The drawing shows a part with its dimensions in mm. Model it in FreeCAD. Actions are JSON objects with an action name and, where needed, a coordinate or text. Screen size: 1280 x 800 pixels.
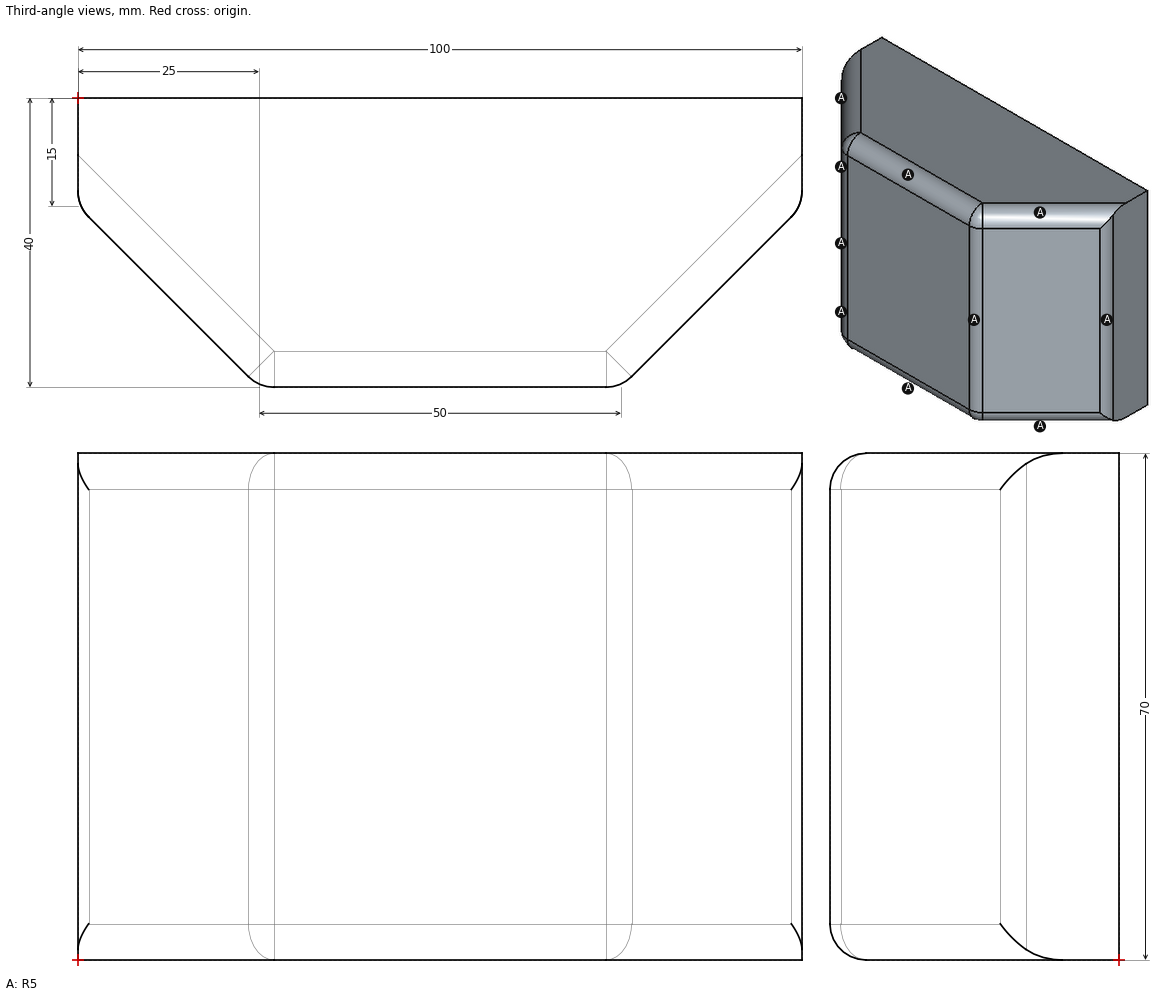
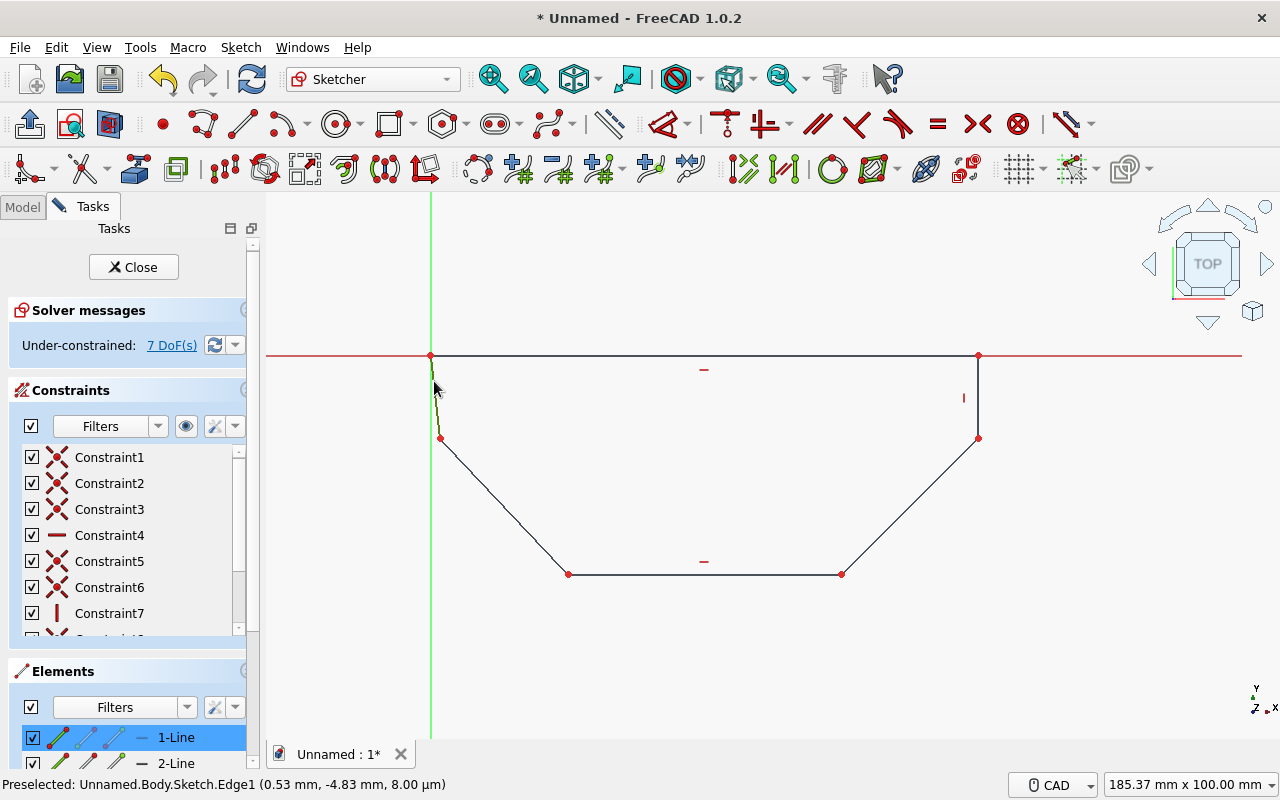
{"action": "left_click", "coordinate": [792, 124]}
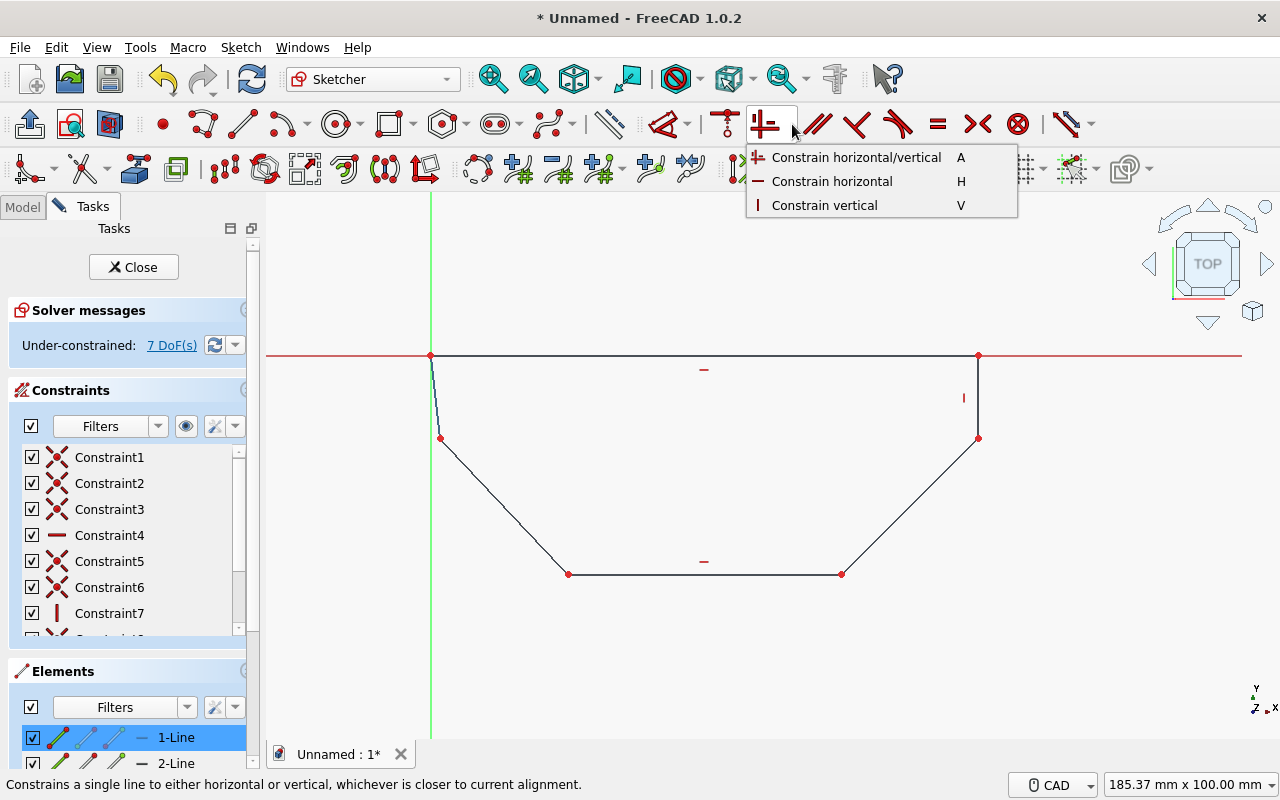
{"action": "left_click", "coordinate": [882, 205]}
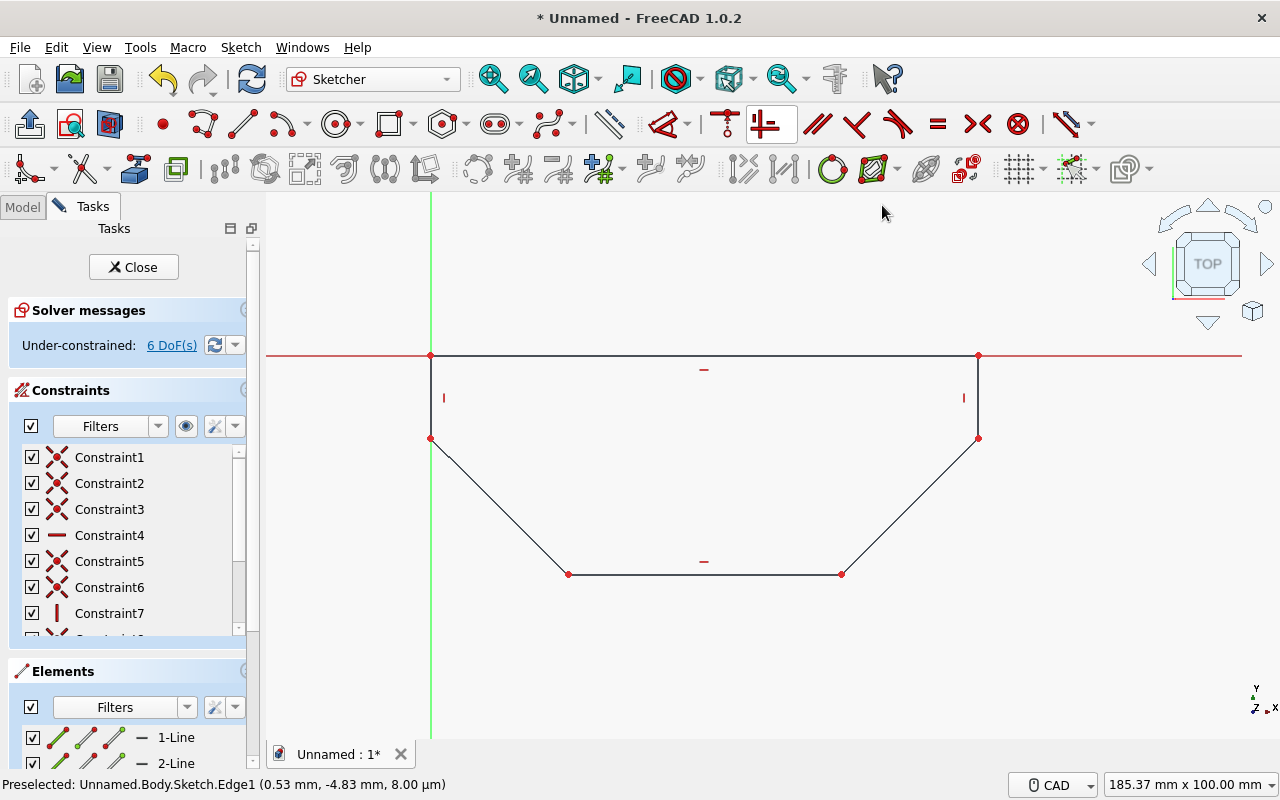
{"action": "left_click", "coordinate": [431, 381]}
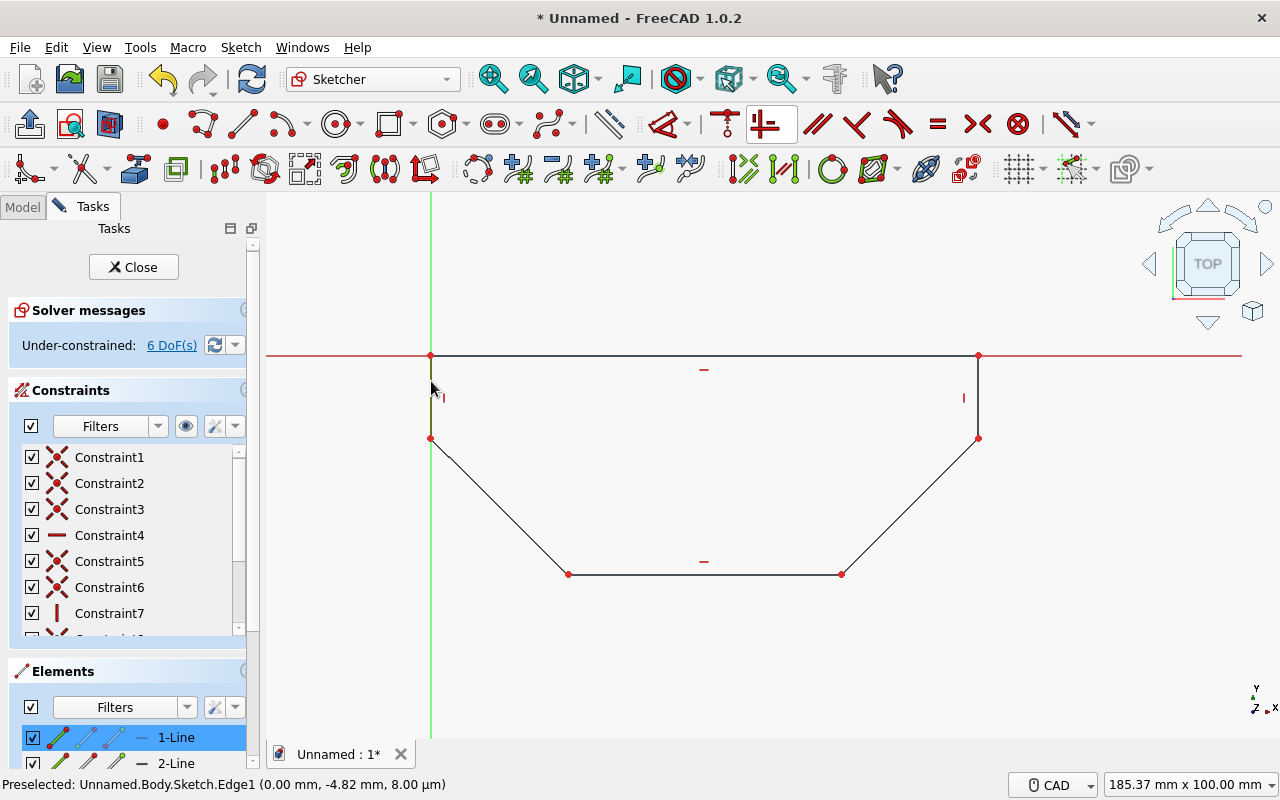
{"action": "key", "text": "i"}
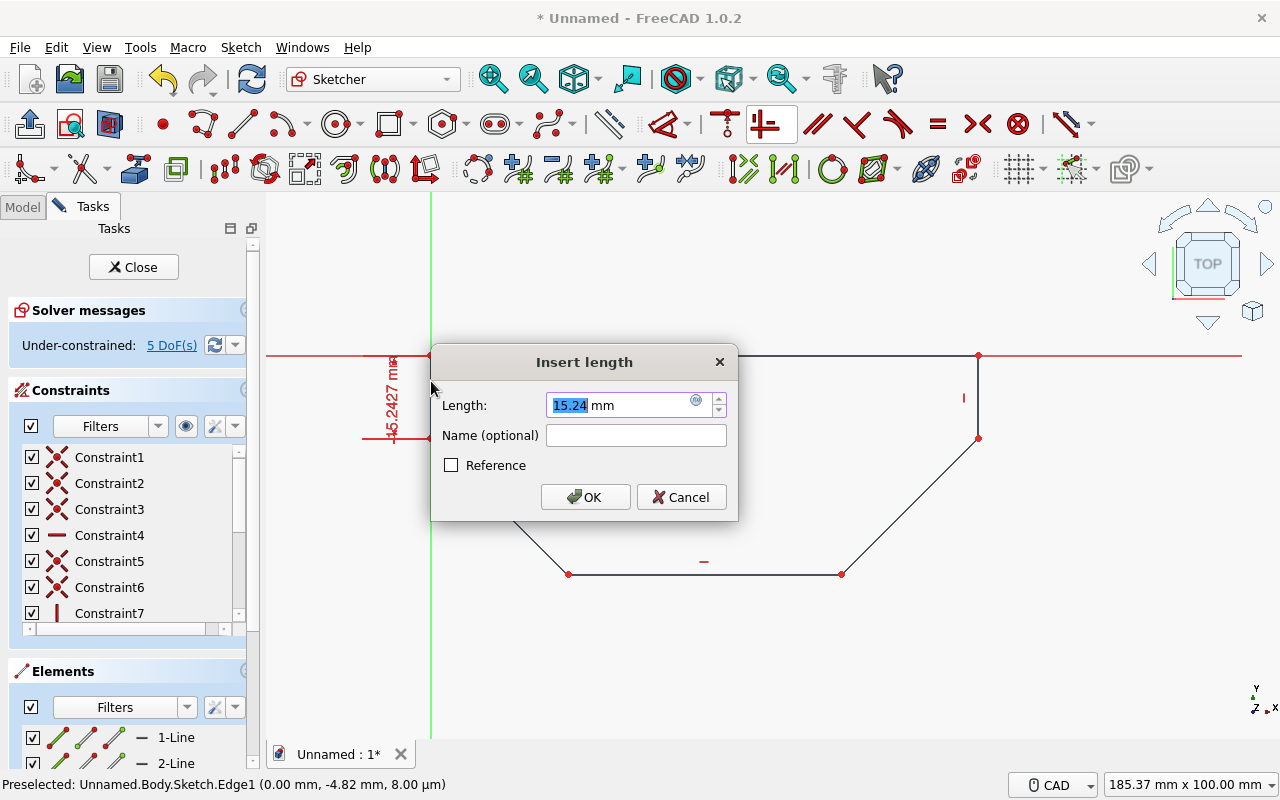
{"action": "type", "text": "15"}
{"action": "key", "text": "Return"}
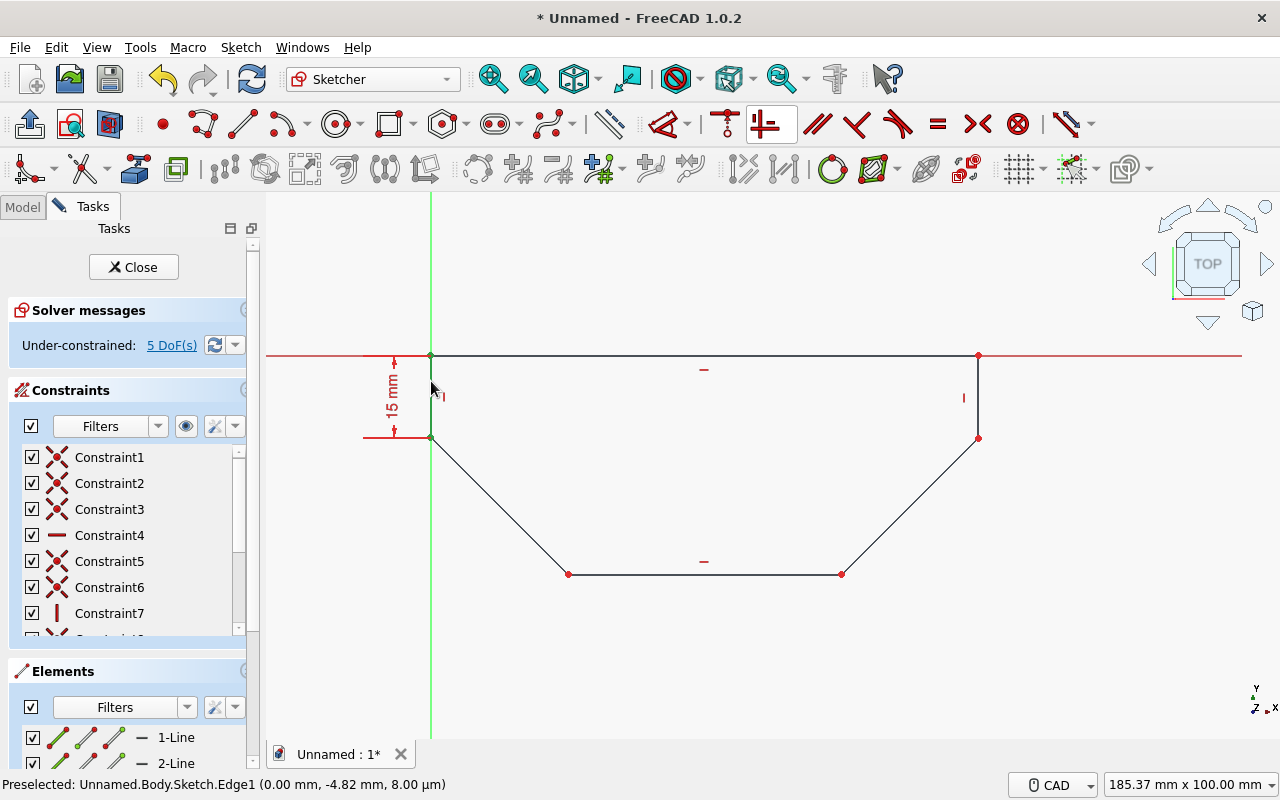
{"action": "left_click", "coordinate": [650, 575]}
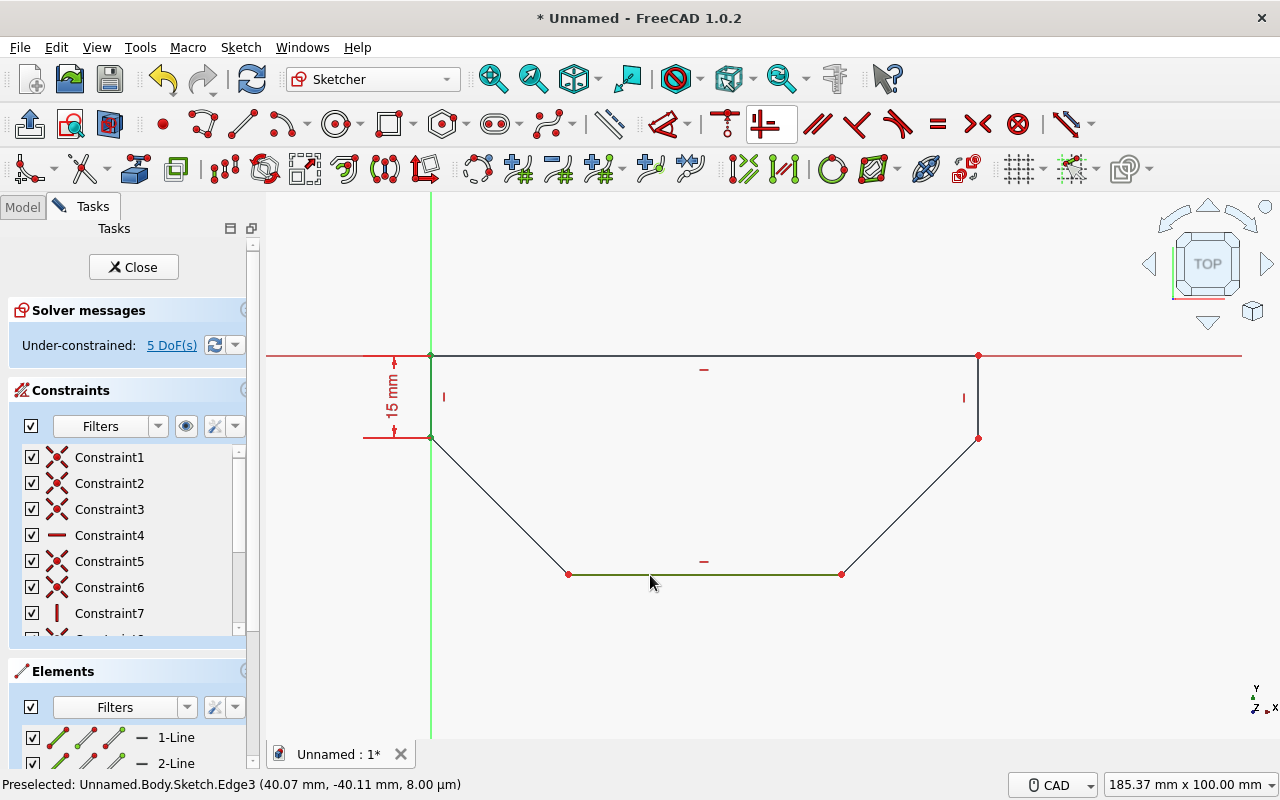
{"action": "key", "text": "l"}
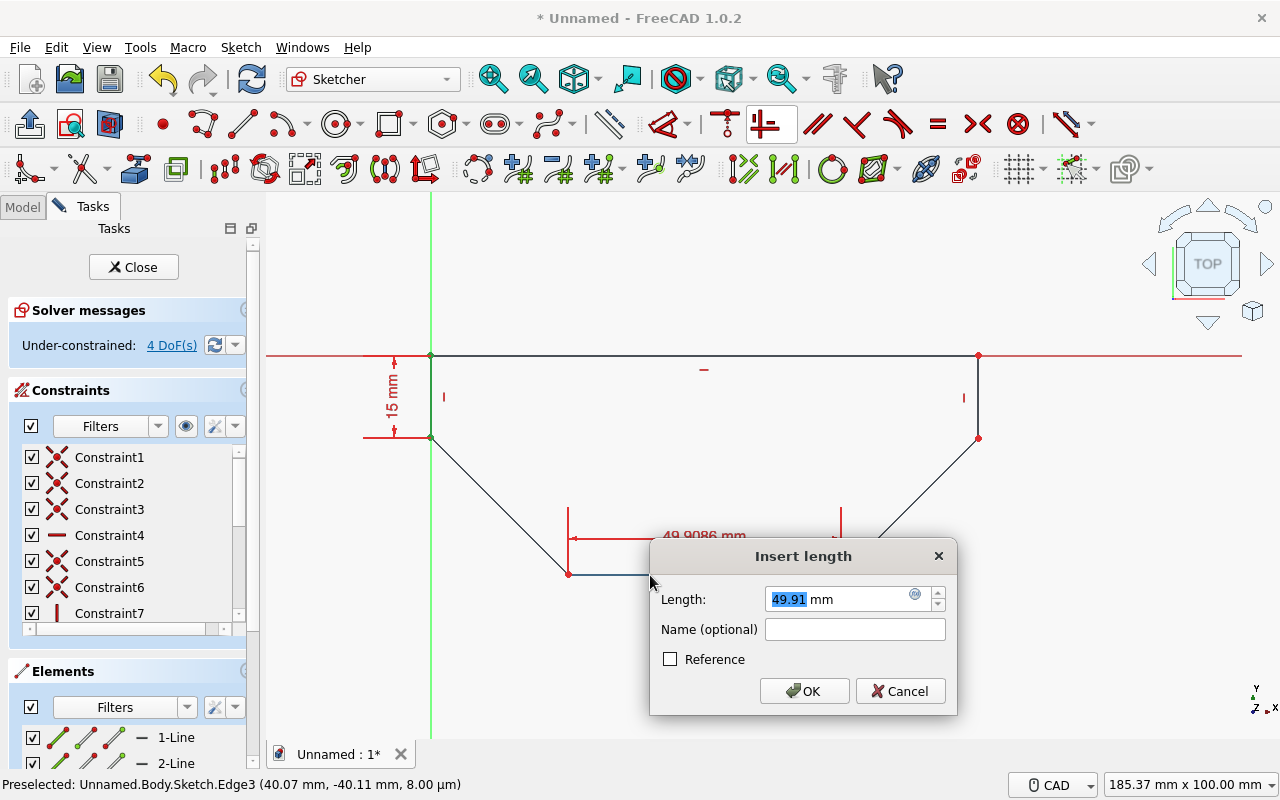
{"action": "type", "text": "50"}
{"action": "key", "text": "Return"}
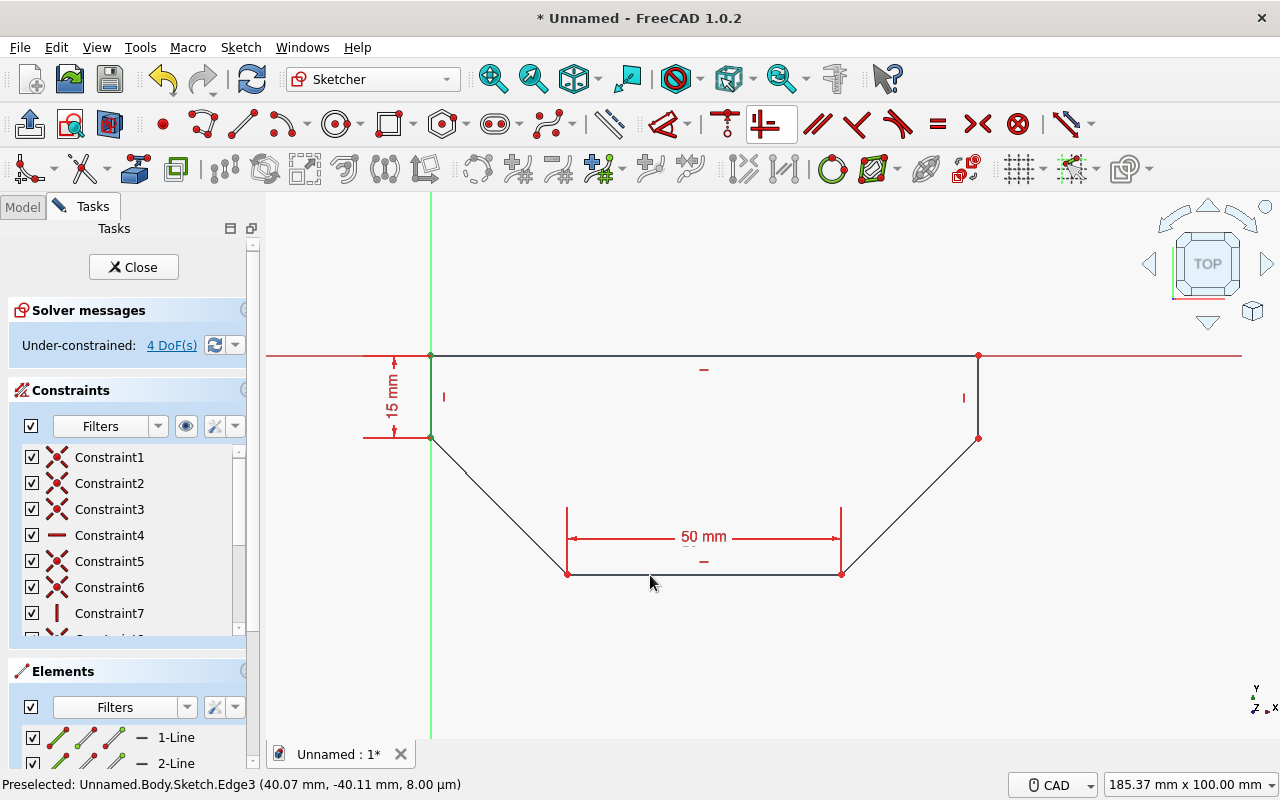
{"action": "left_click", "coordinate": [978, 414]}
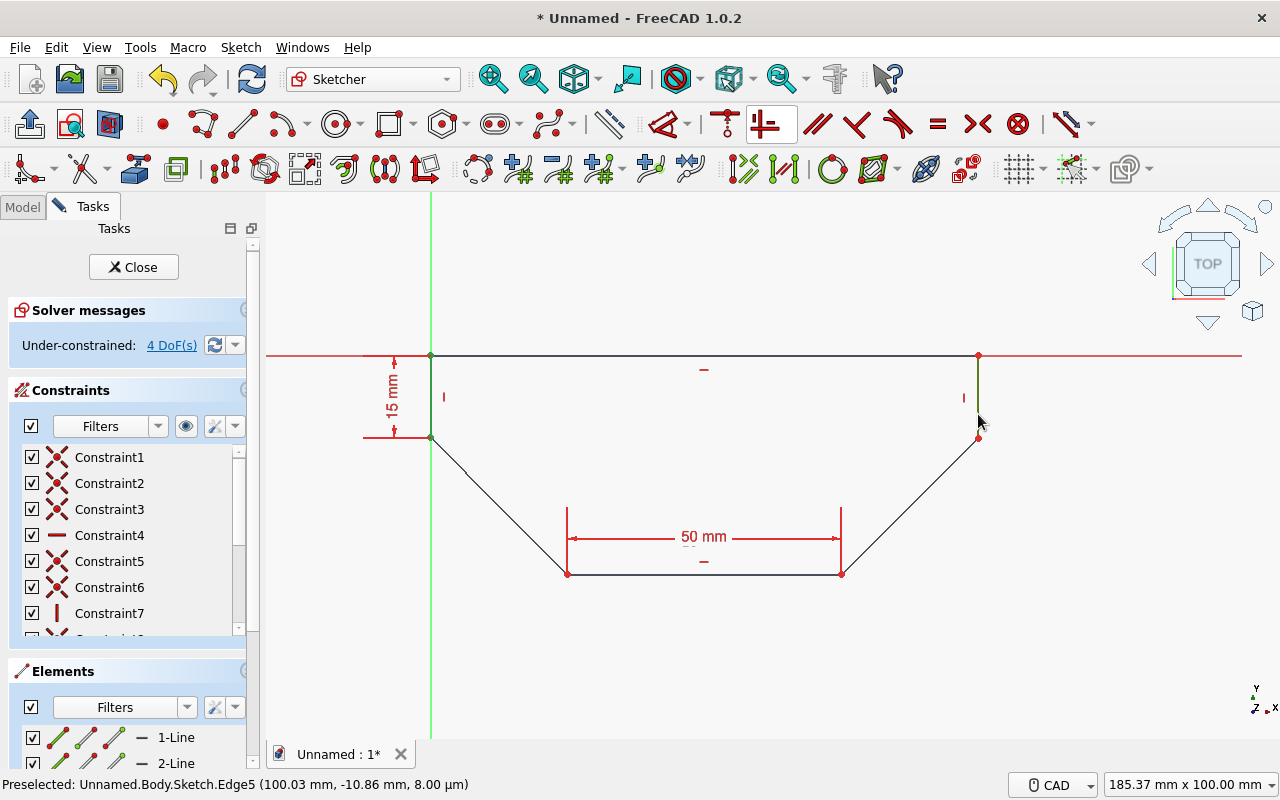
{"action": "left_click", "coordinate": [690, 124]}